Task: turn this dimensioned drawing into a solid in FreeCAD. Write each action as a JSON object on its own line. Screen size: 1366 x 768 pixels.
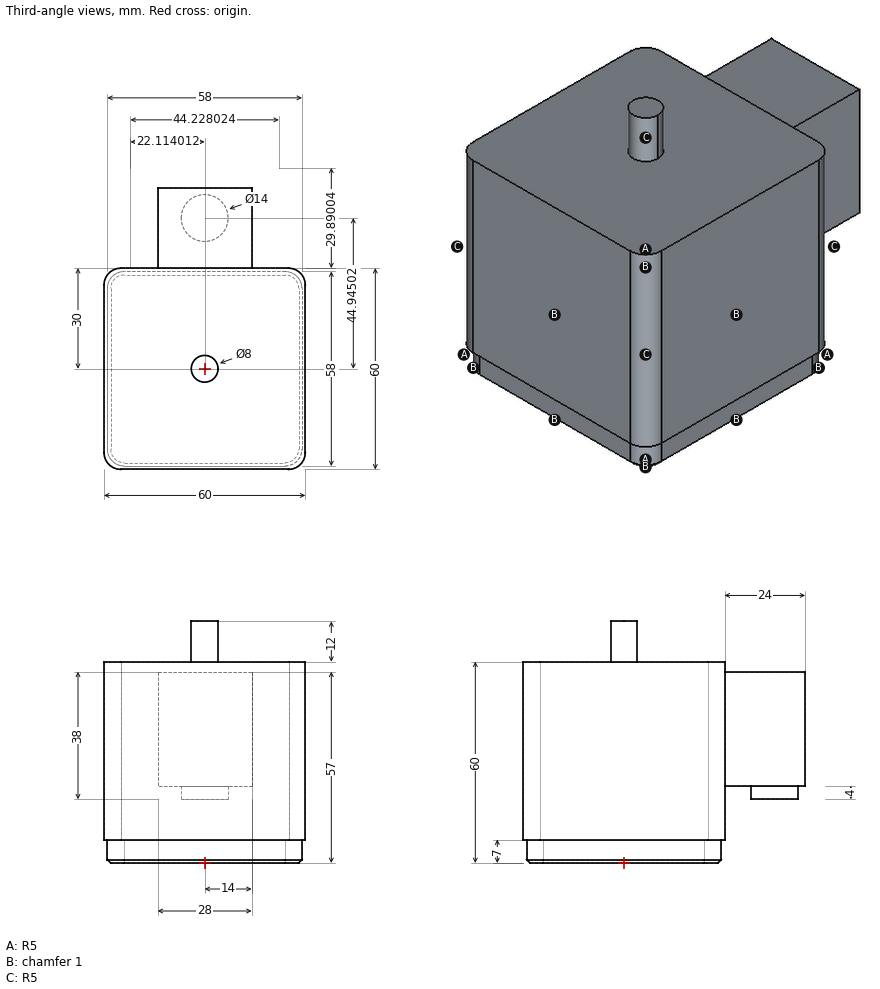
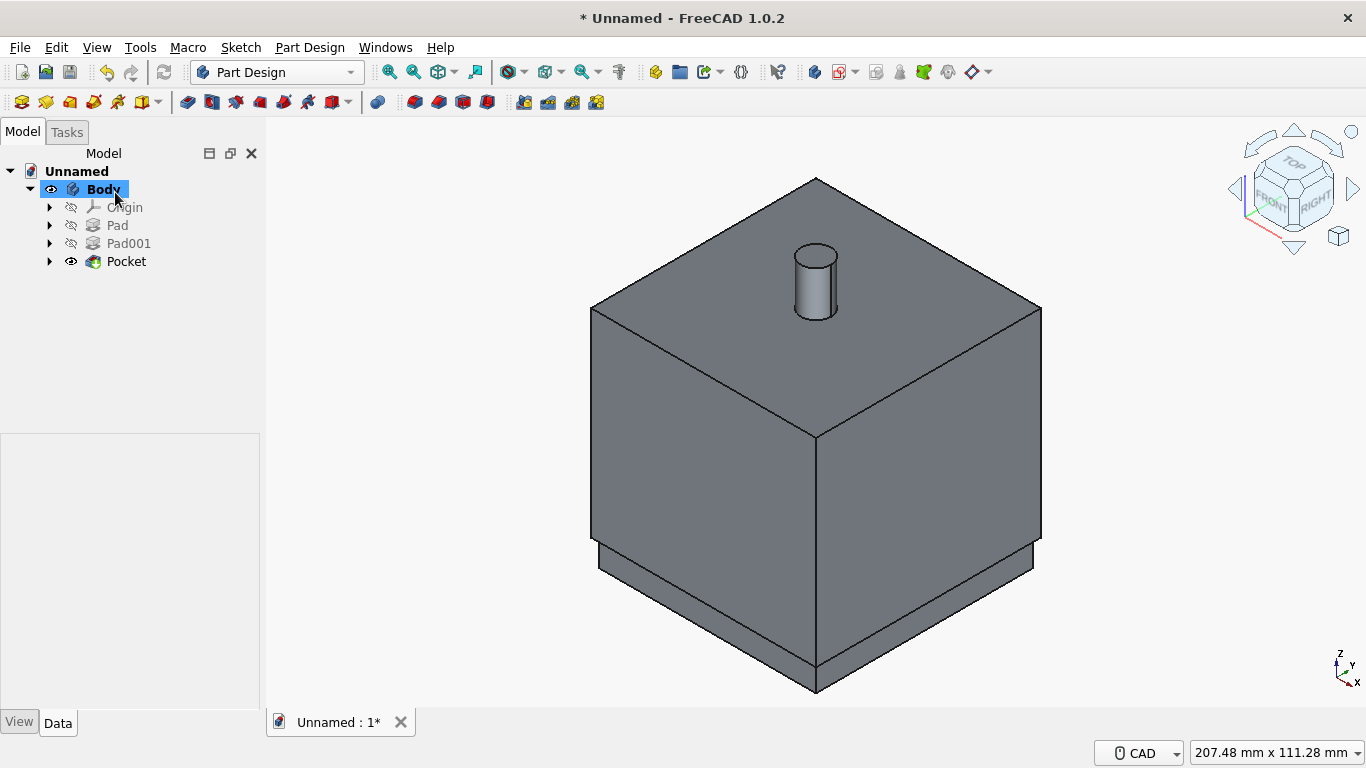
{"action": "left_click", "coordinate": [816, 677]}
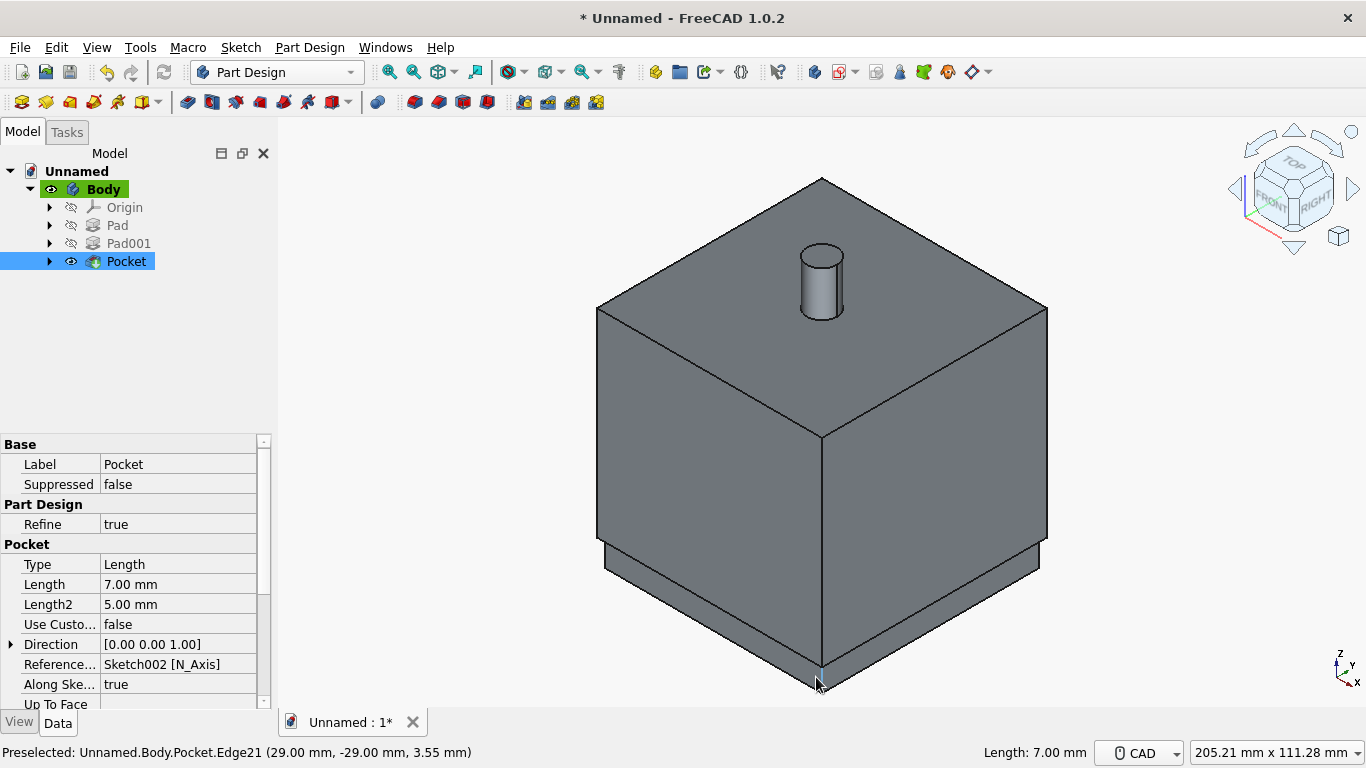
{"action": "key", "text": "2"}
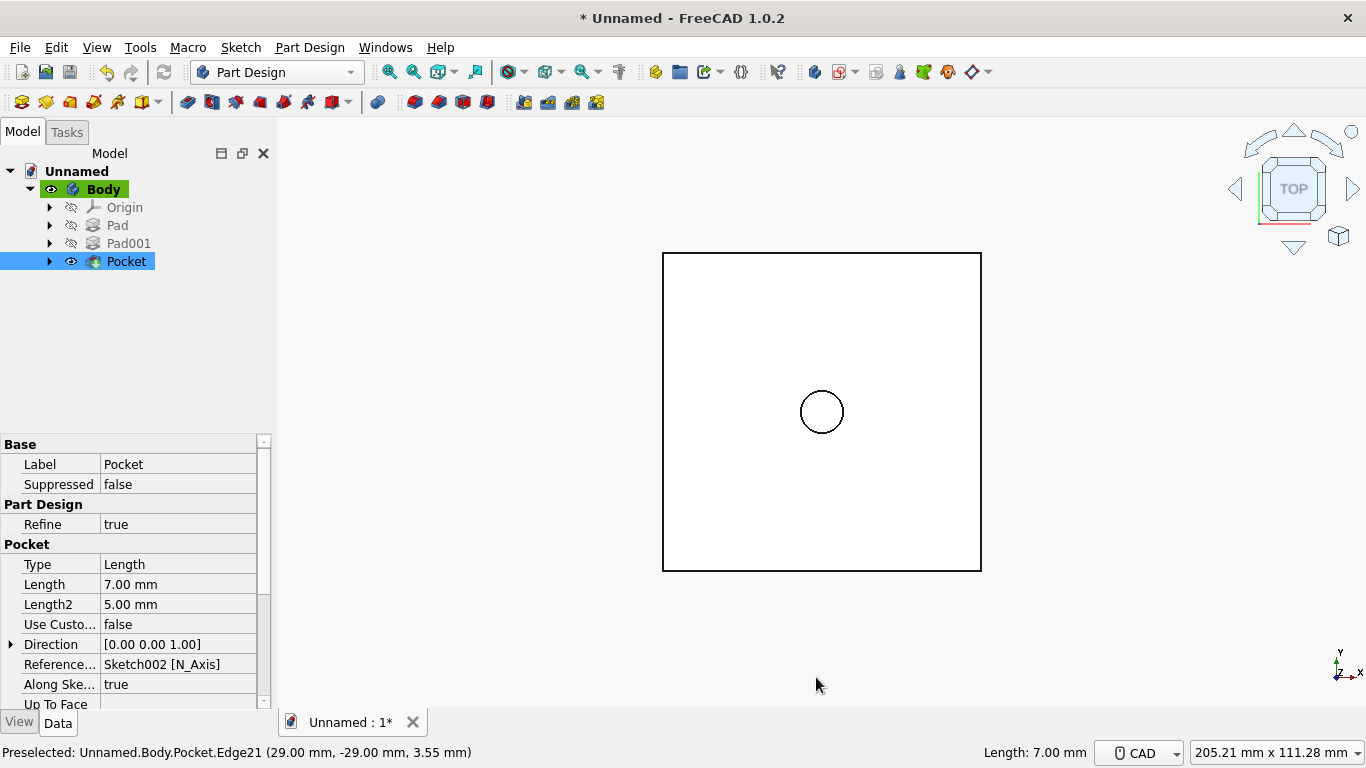
{"action": "key", "text": "1"}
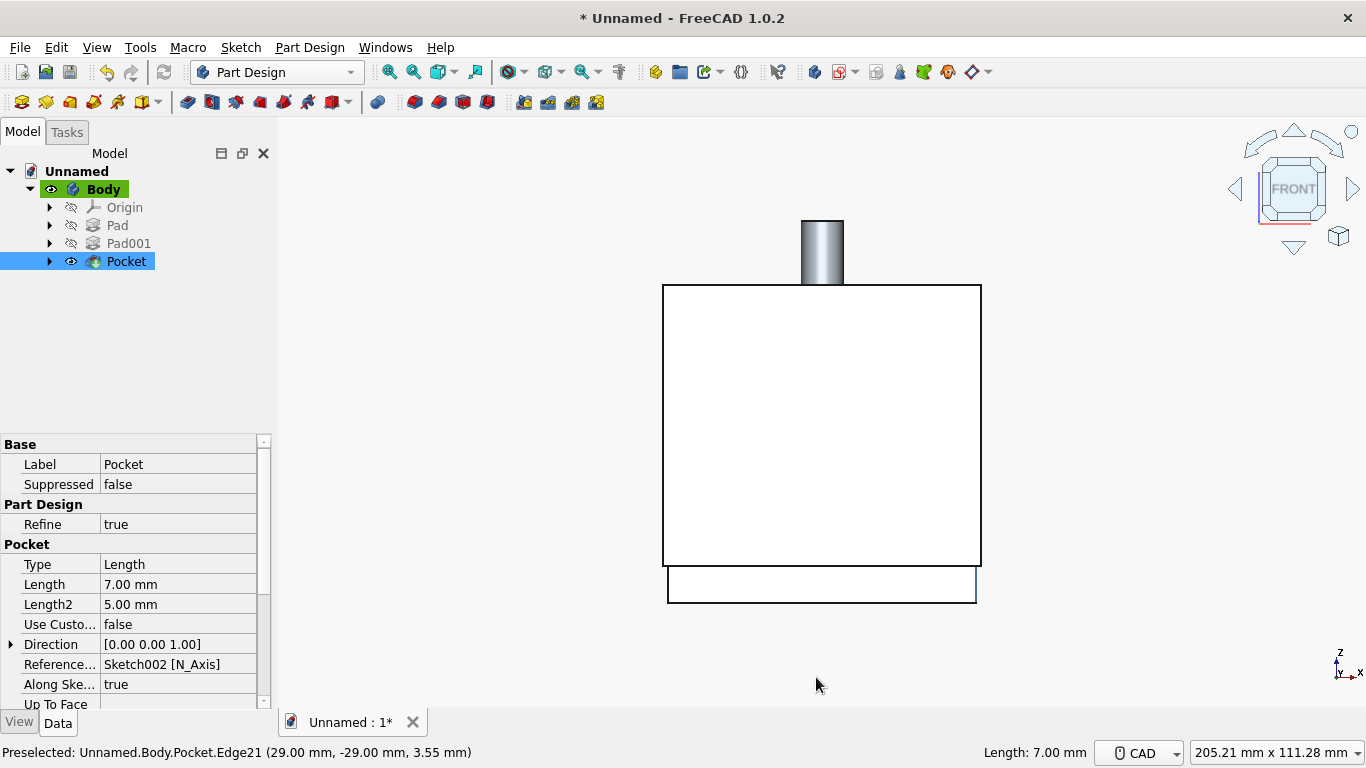
{"action": "left_click", "coordinate": [668, 583], "text": "ctrl"}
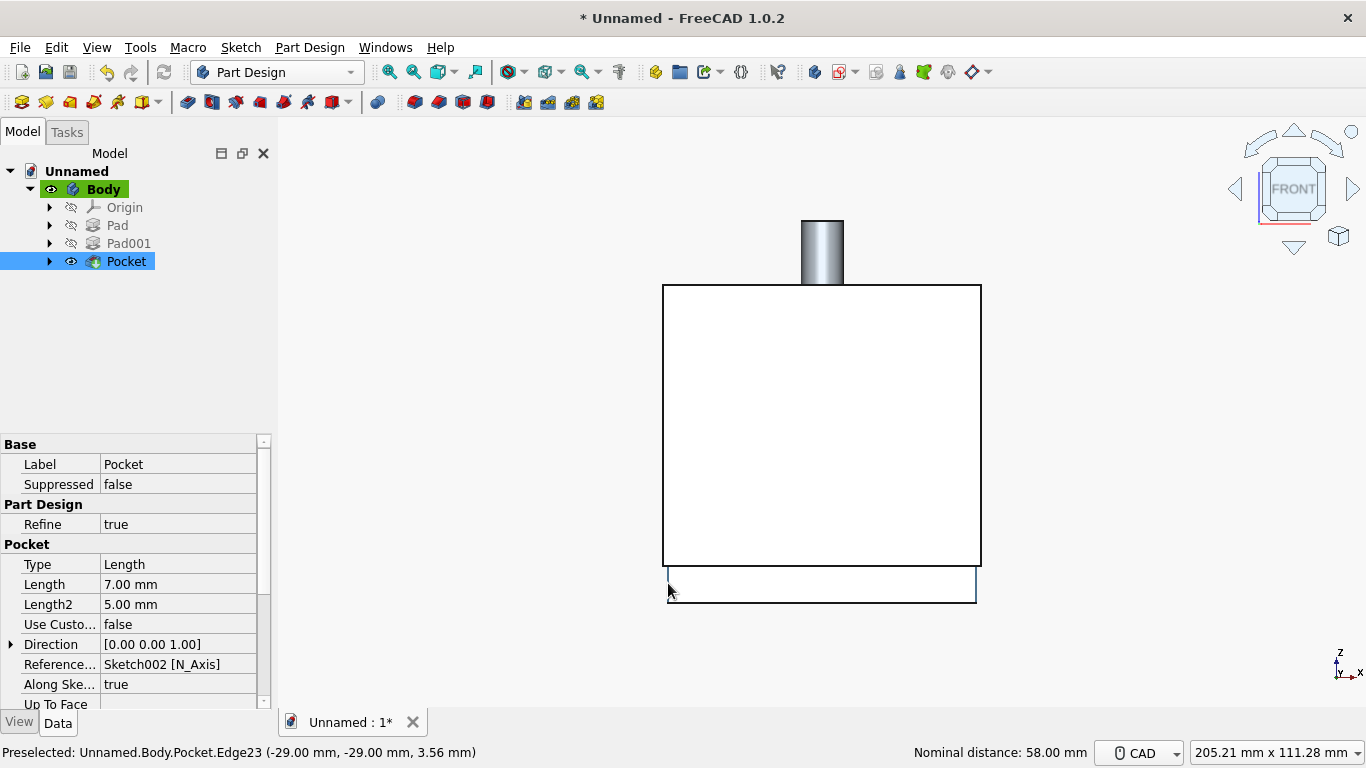
{"action": "key", "text": "3"}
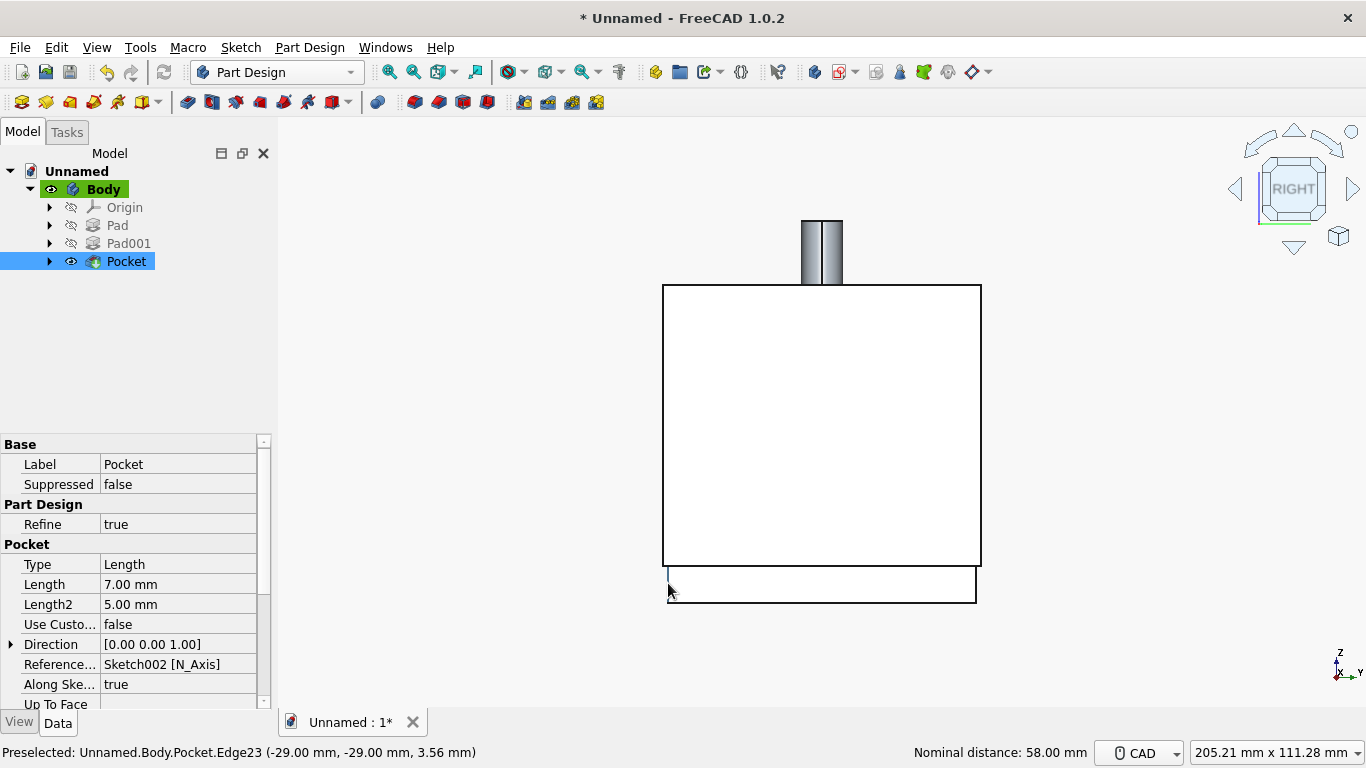
{"action": "left_click", "coordinate": [976, 583], "text": "ctrl"}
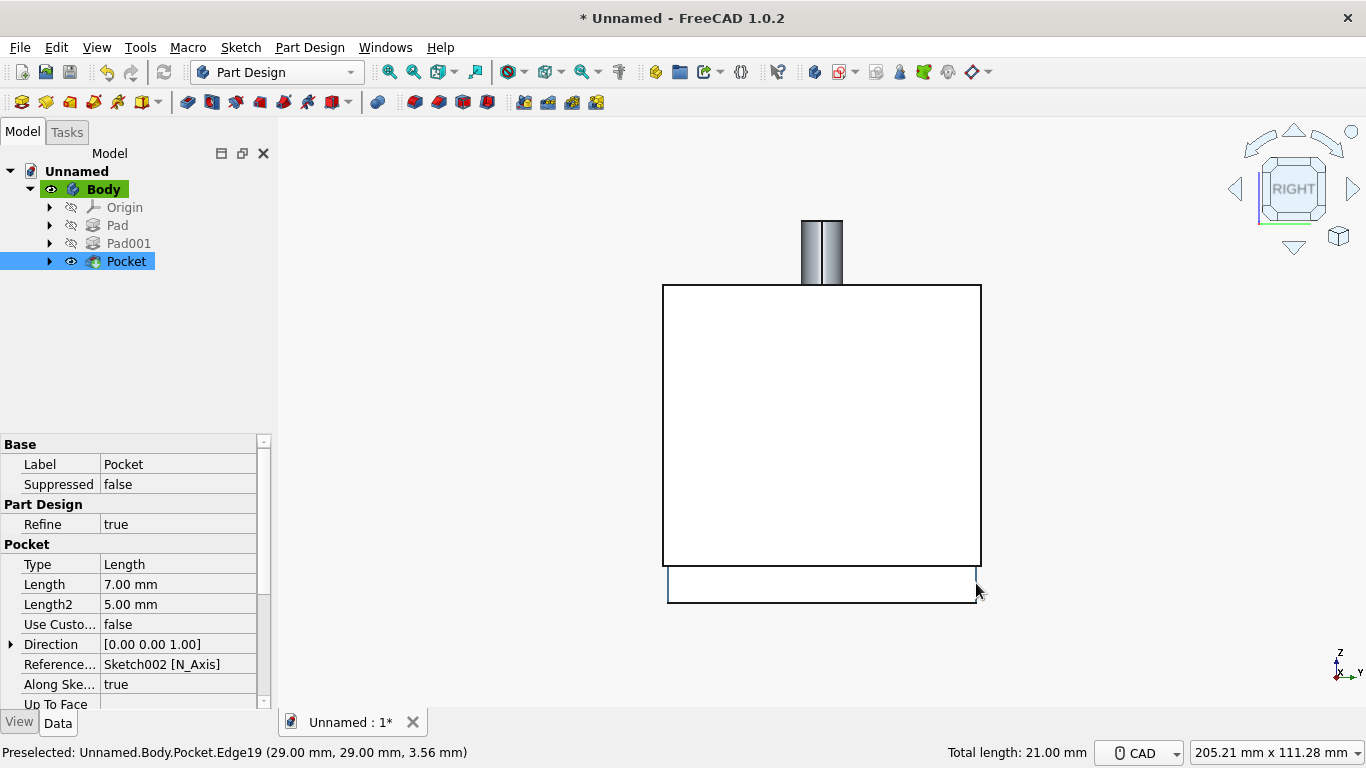
{"action": "key", "text": "5"}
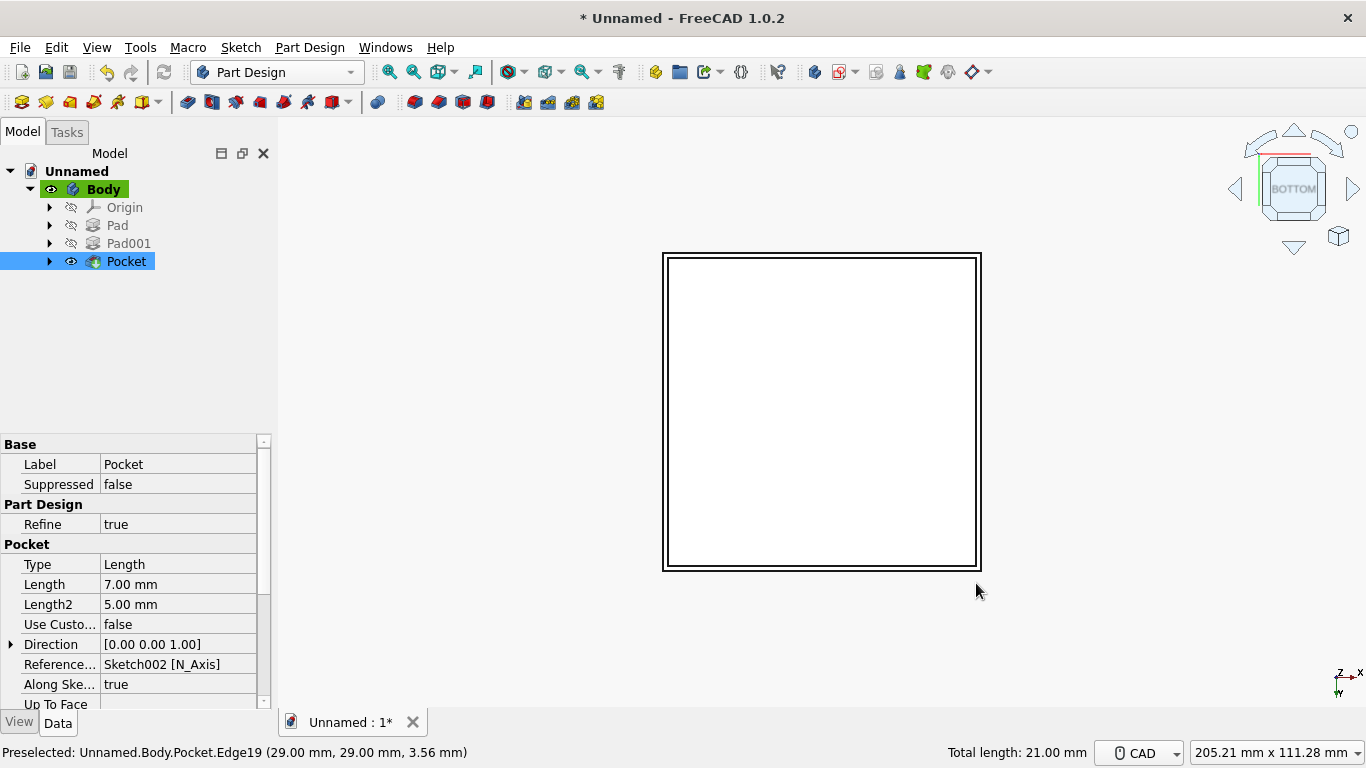
{"action": "key", "text": "4"}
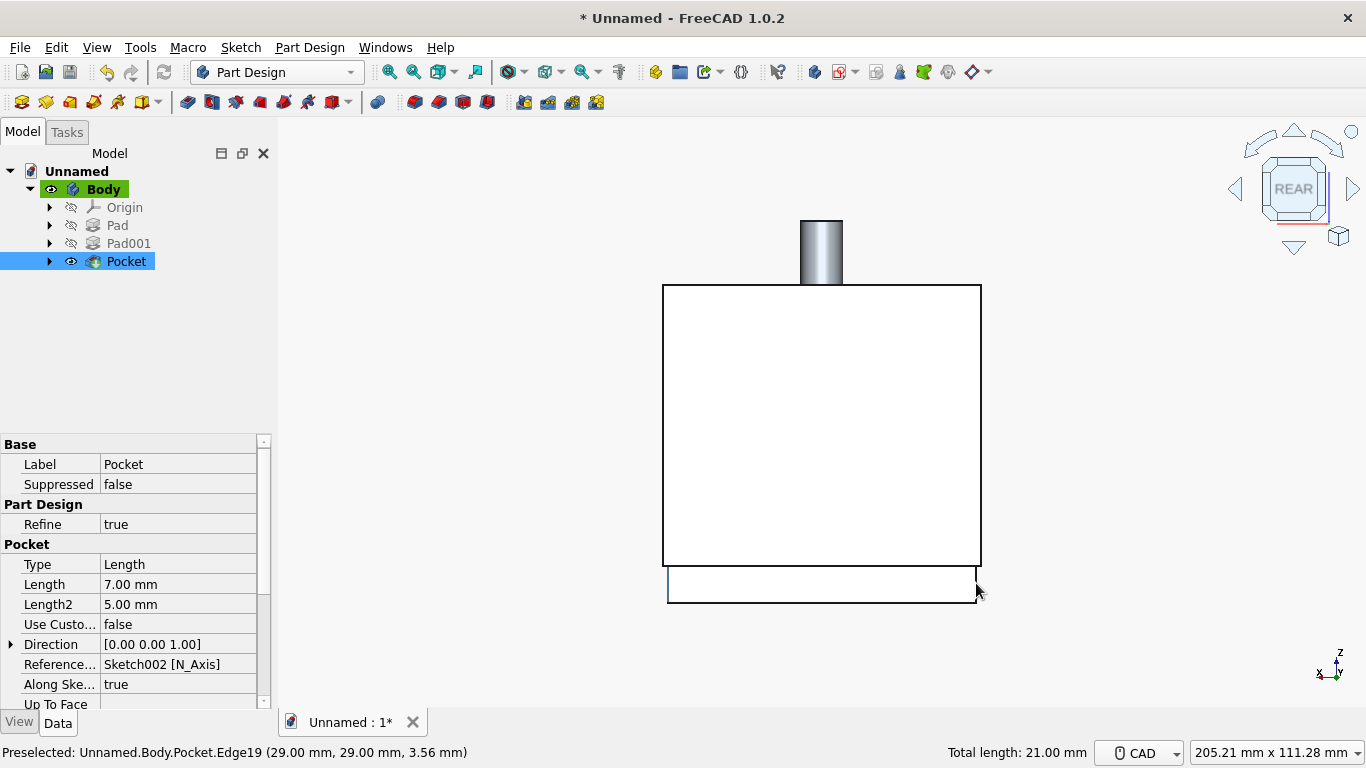
{"action": "left_click", "coordinate": [976, 583], "text": "ctrl"}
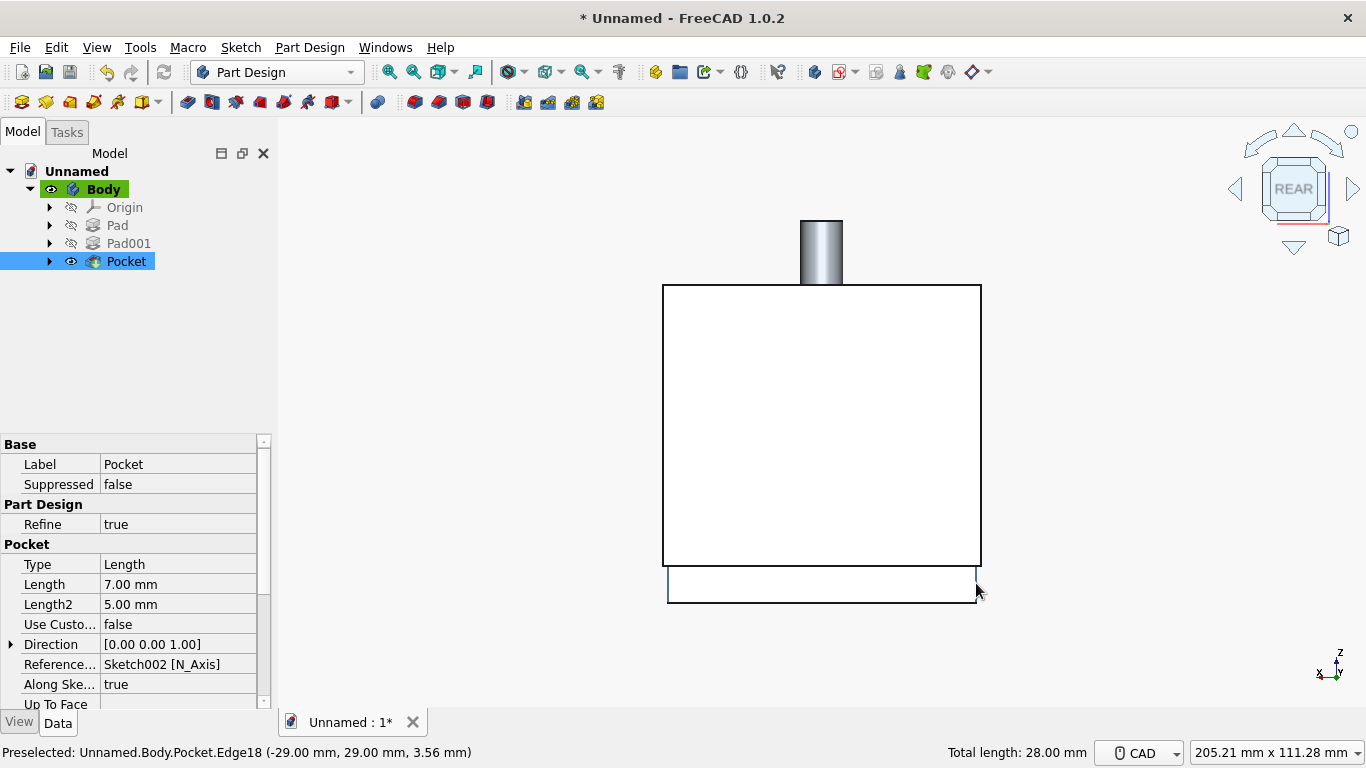
{"action": "left_click", "coordinate": [416, 102]}